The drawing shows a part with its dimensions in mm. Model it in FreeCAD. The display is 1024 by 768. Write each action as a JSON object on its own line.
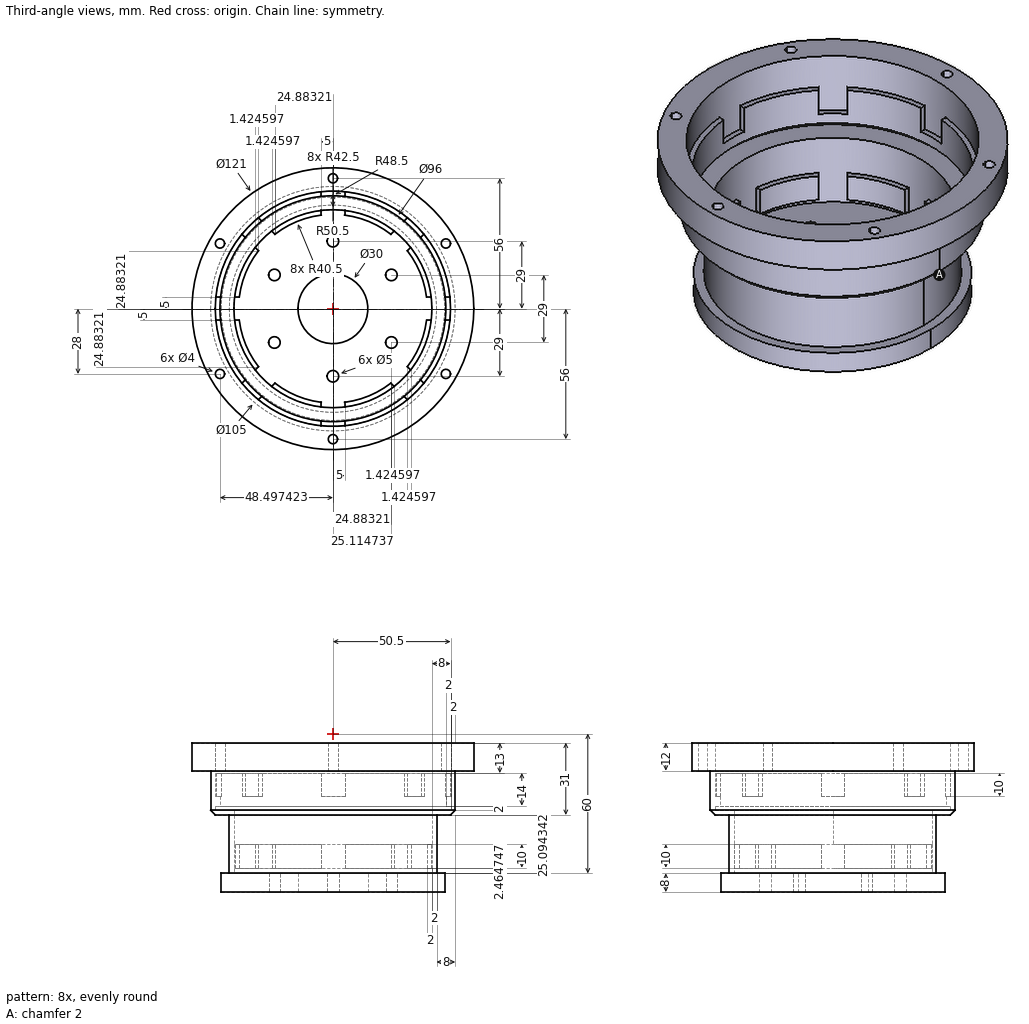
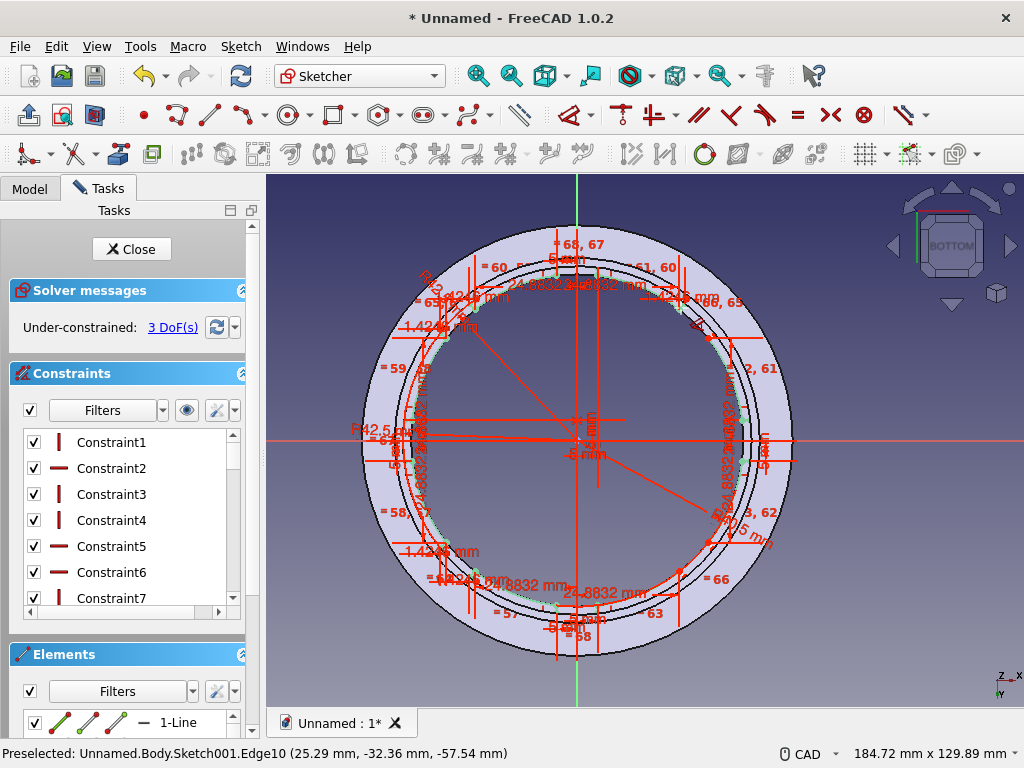
{"action": "scroll", "coordinate": [713, 335], "scroll_direction": "up", "scroll_amount": 10}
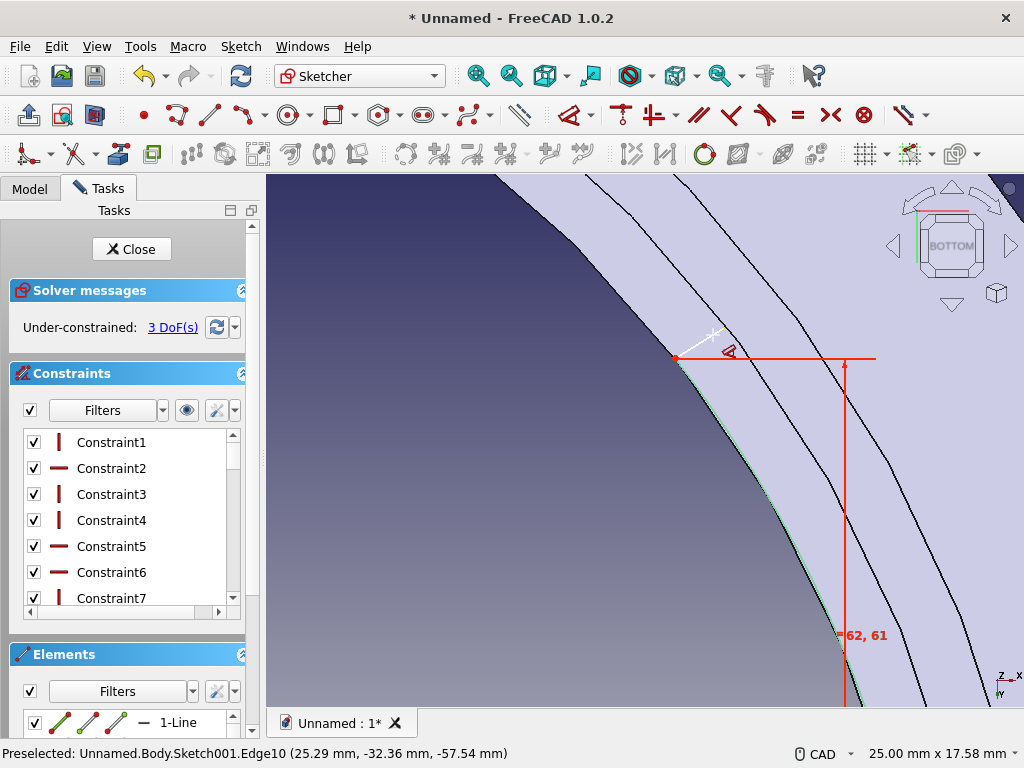
{"action": "left_click", "coordinate": [711, 336]}
{"action": "left_click", "coordinate": [719, 292]}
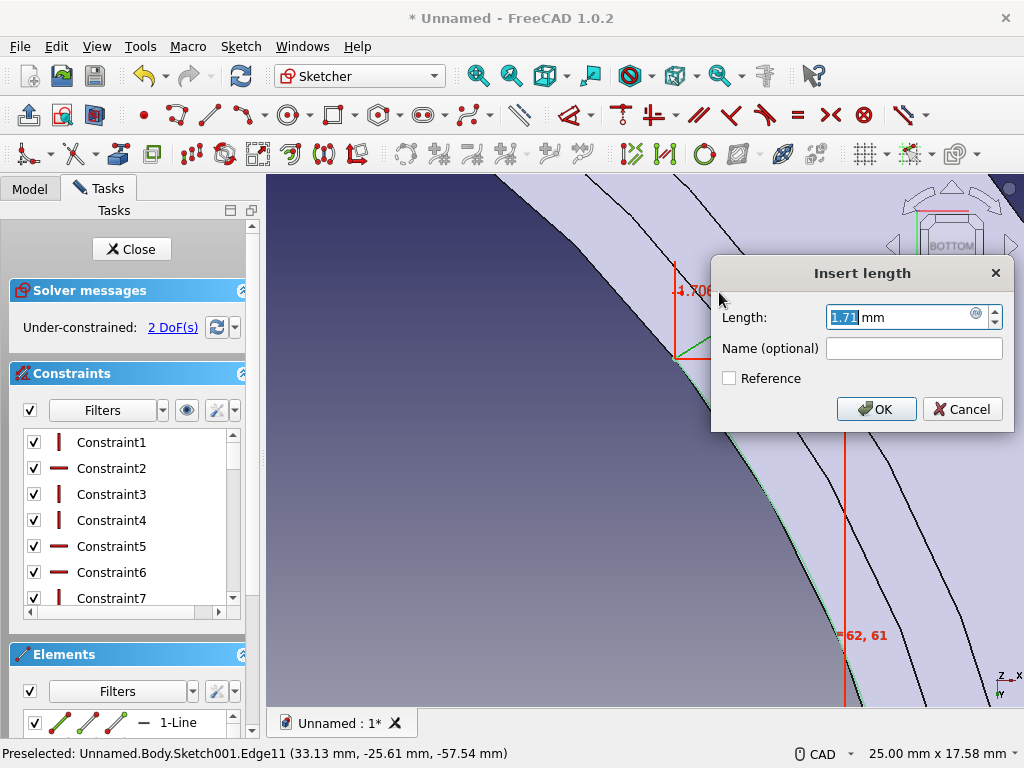
{"action": "type", "text": "1.424597"}
{"action": "key", "text": "Return"}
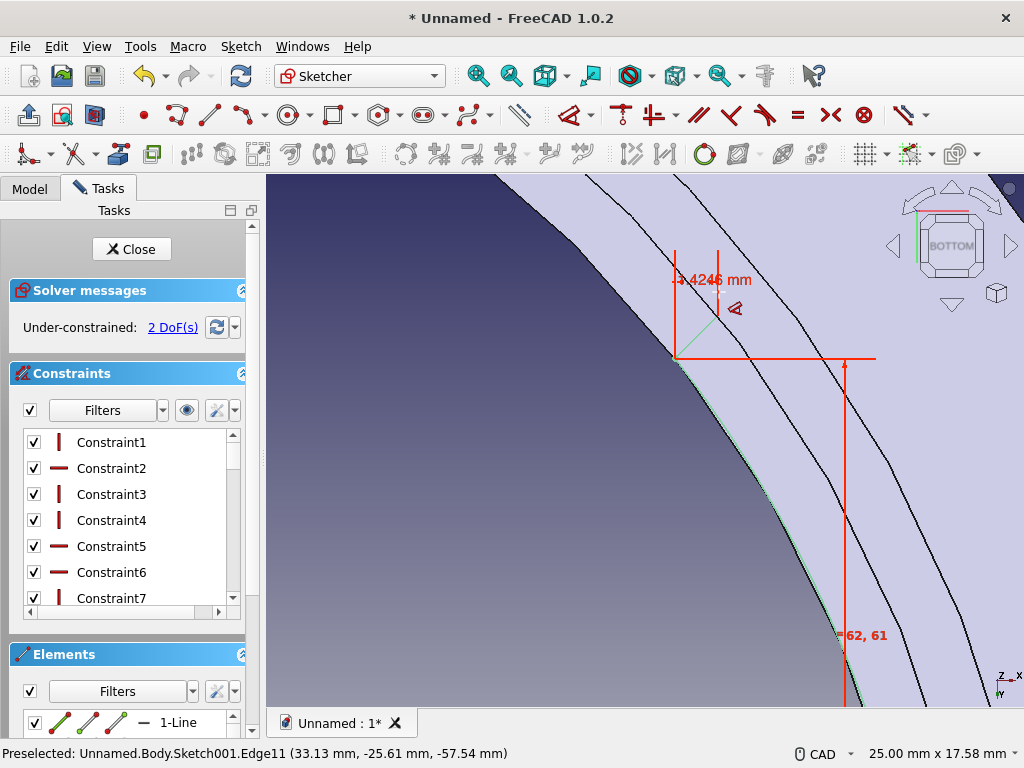
{"action": "scroll", "coordinate": [713, 335], "scroll_direction": "down", "scroll_amount": 10}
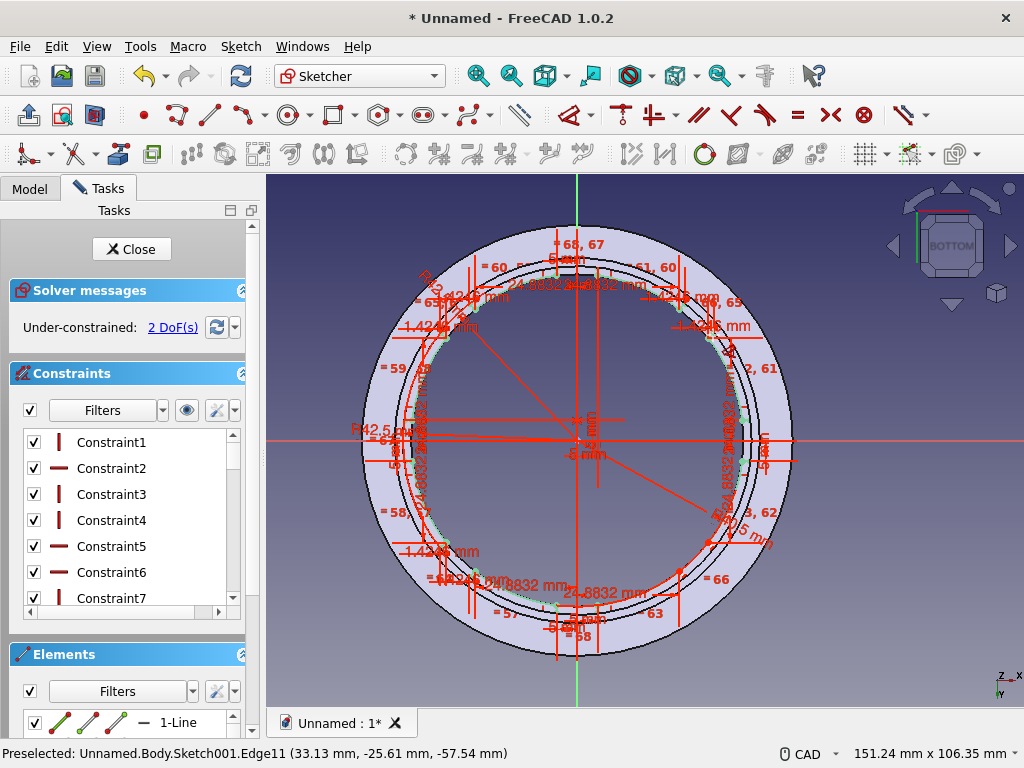
{"action": "scroll", "coordinate": [710, 545], "scroll_direction": "up", "scroll_amount": 10}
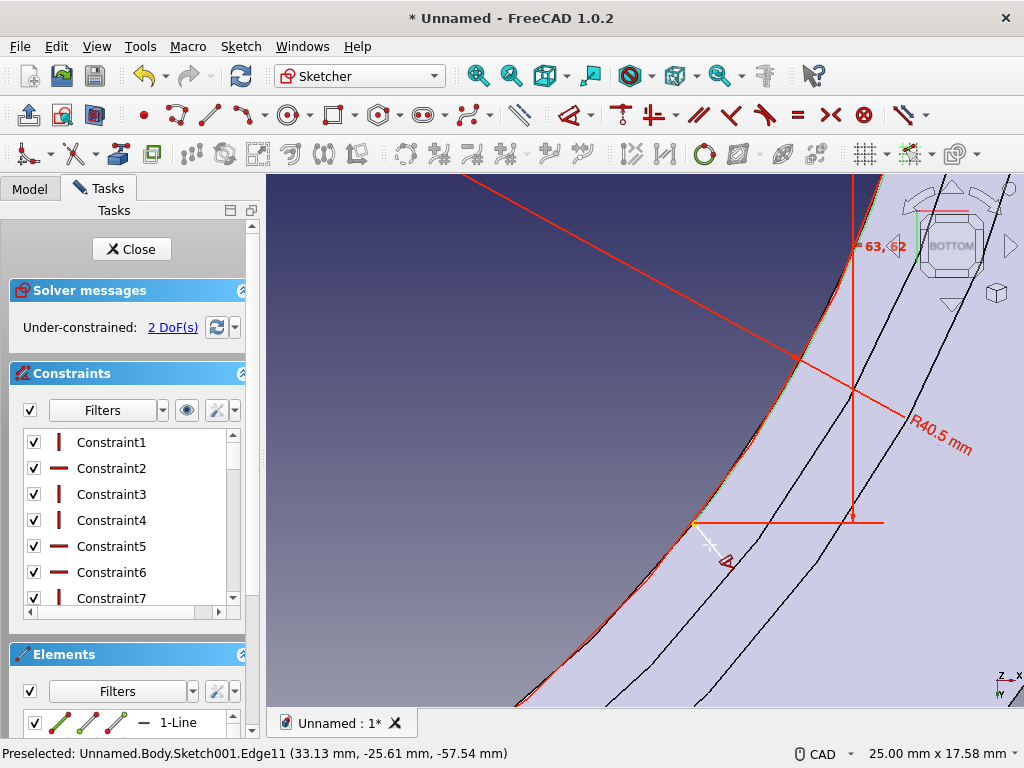
{"action": "left_click", "coordinate": [706, 538]}
{"action": "left_click", "coordinate": [723, 606]}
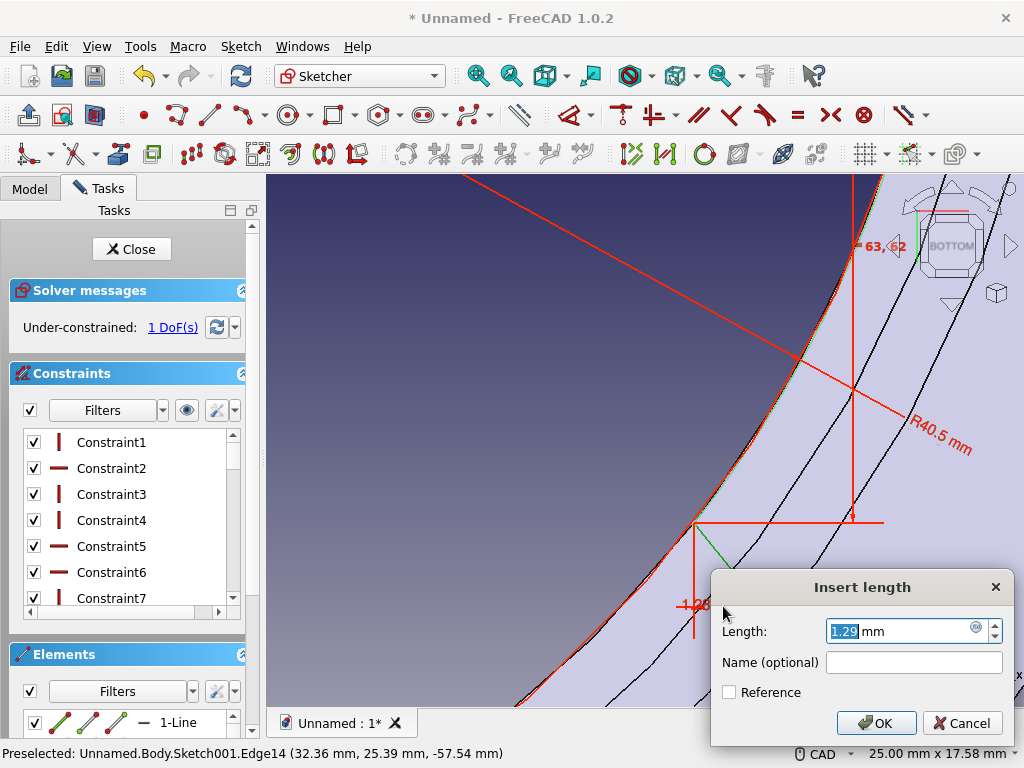
{"action": "type", "text": "1.424597"}
{"action": "key", "text": "Return"}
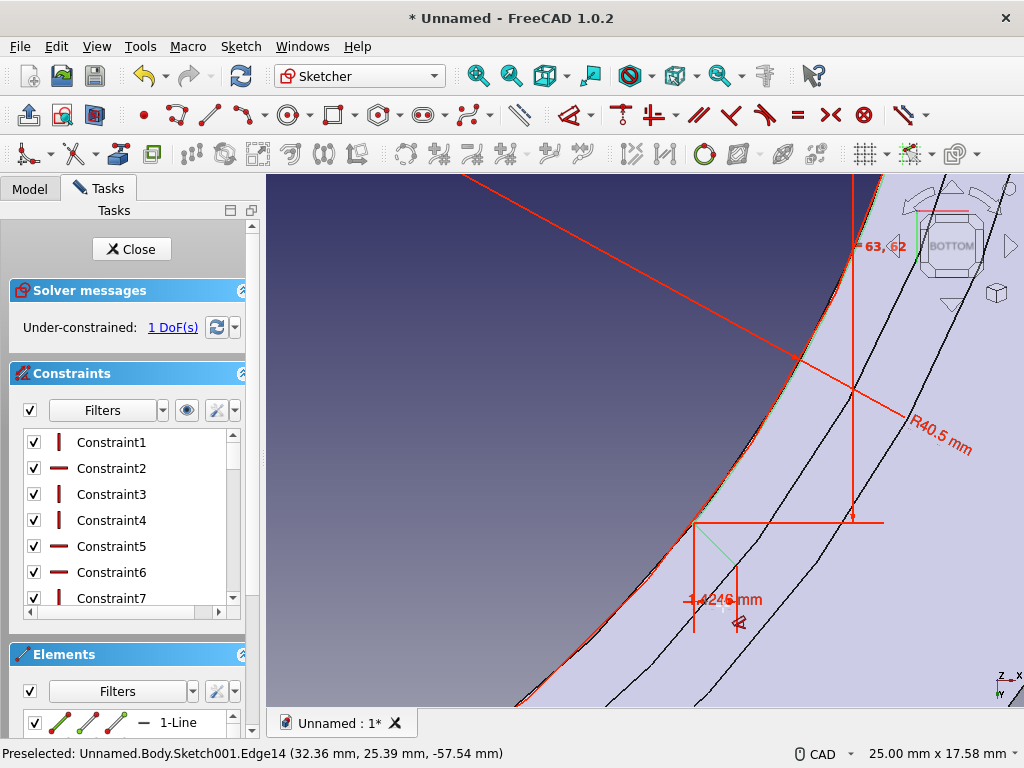
{"action": "scroll", "coordinate": [710, 546], "scroll_direction": "down", "scroll_amount": 10}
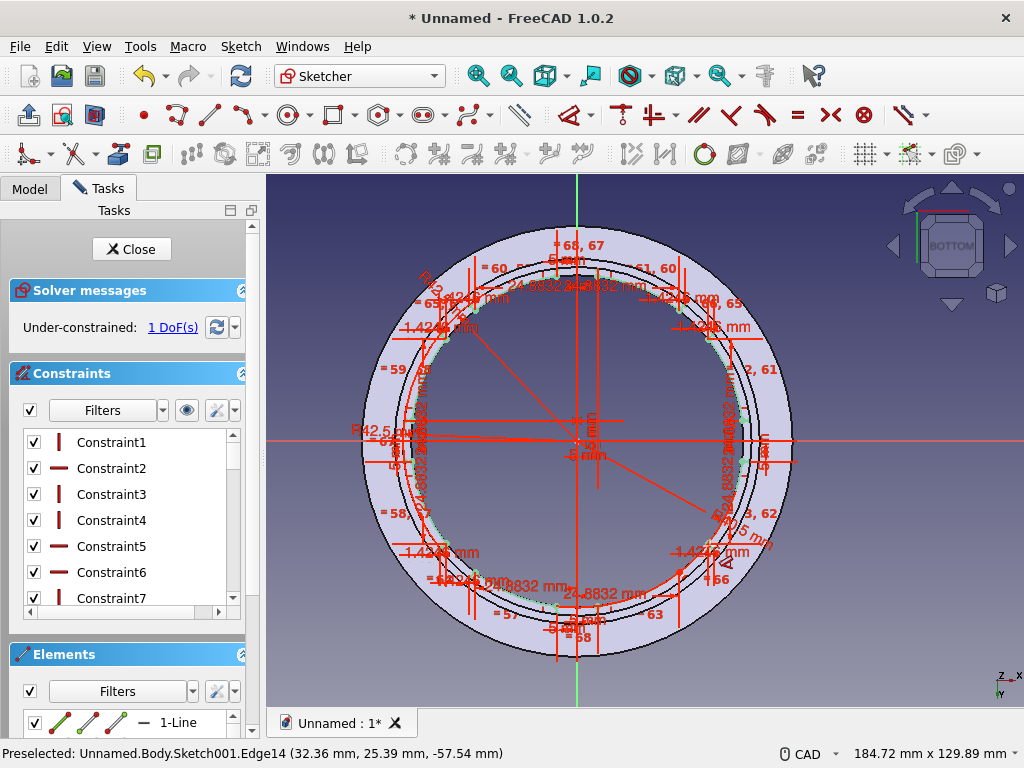
{"action": "scroll", "coordinate": [684, 577], "scroll_direction": "up", "scroll_amount": 10}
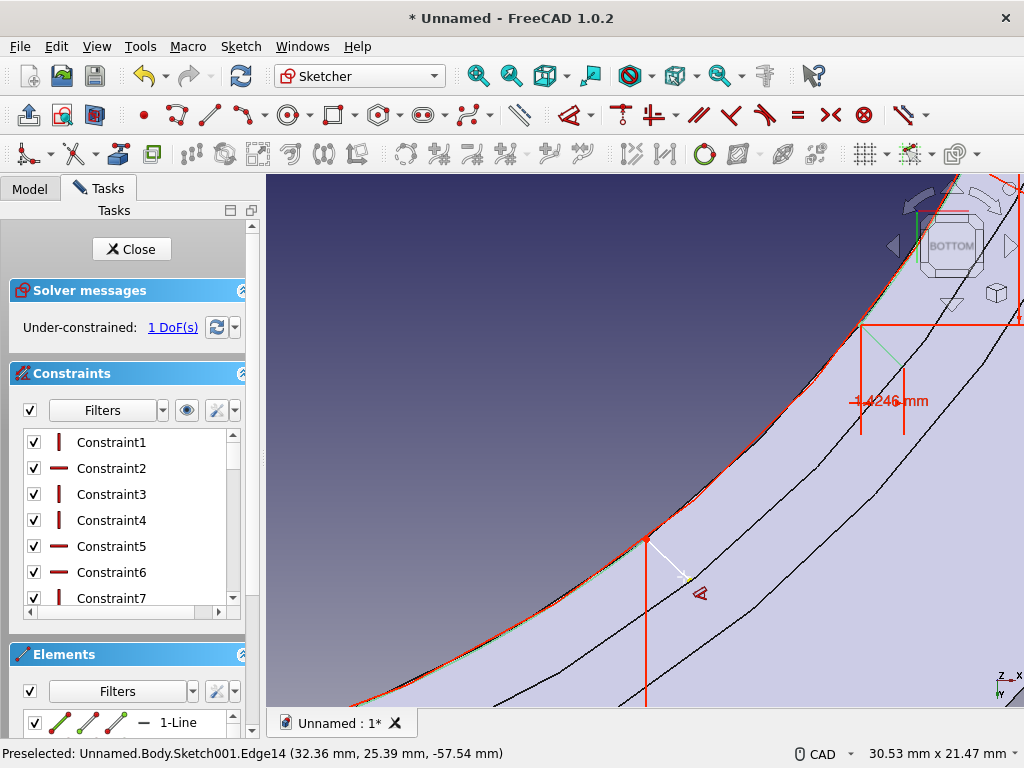
{"action": "left_click", "coordinate": [677, 569]}
{"action": "left_click", "coordinate": [669, 615]}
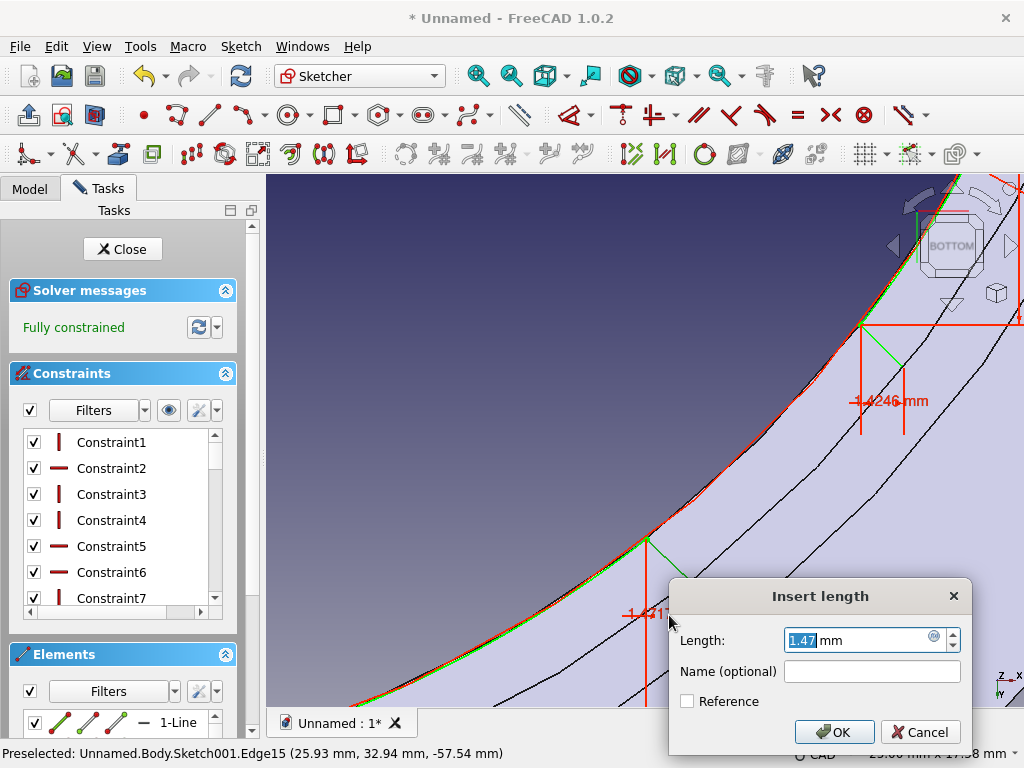
{"action": "type", "text": "1.424597"}
{"action": "key", "text": "Return"}
{"action": "key", "text": "Escape"}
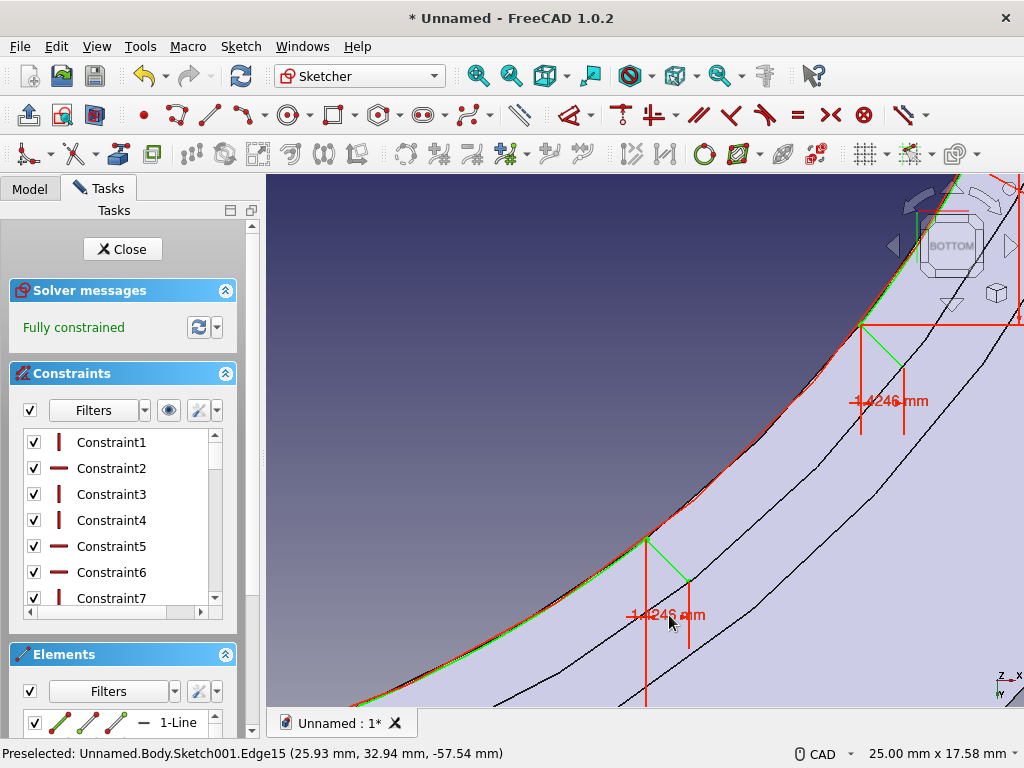
{"action": "left_click", "coordinate": [123, 249]}